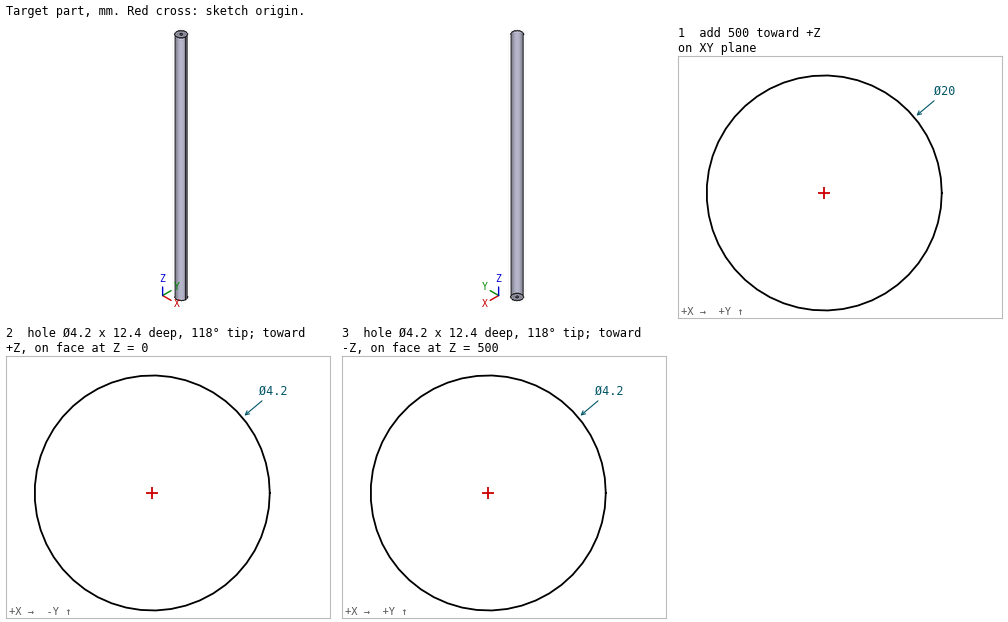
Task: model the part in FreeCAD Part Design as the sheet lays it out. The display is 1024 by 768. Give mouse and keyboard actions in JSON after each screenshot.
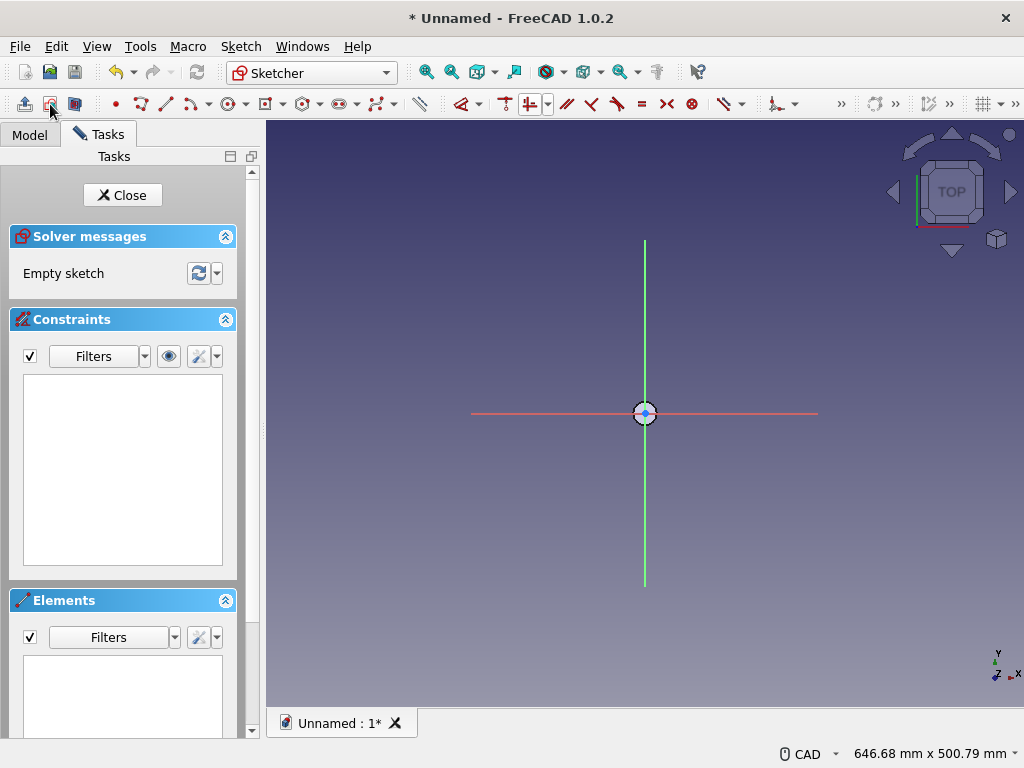
{"action": "scroll", "coordinate": [649, 414], "scroll_direction": "up", "scroll_amount": 15}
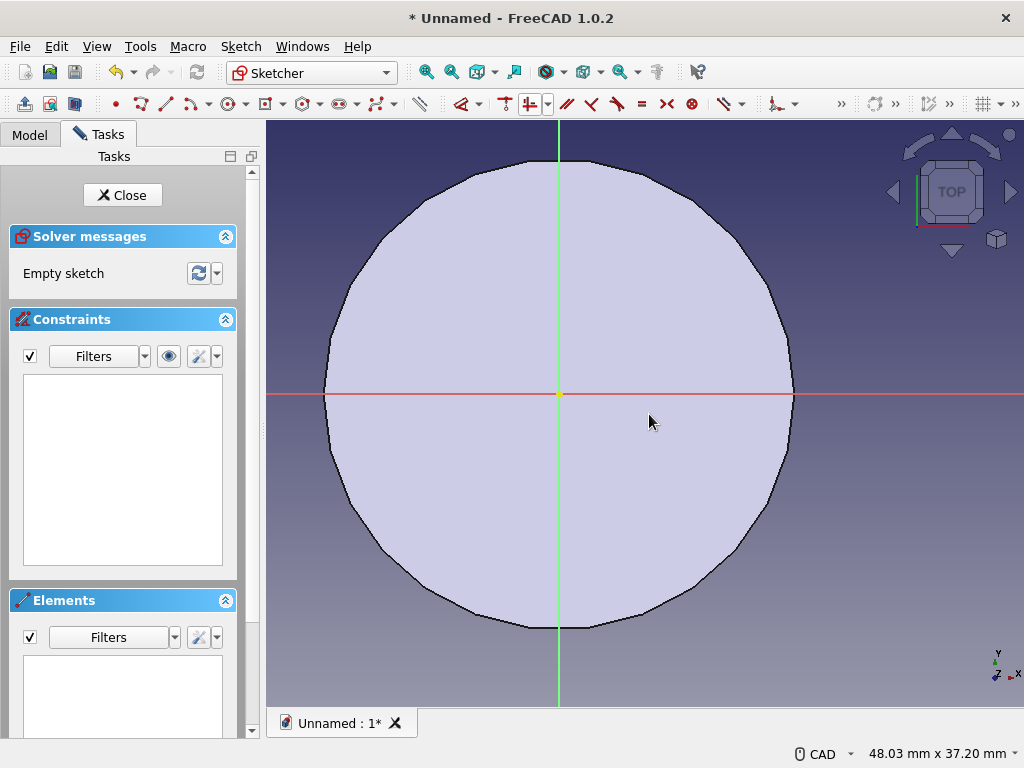
{"action": "scroll", "coordinate": [553, 388], "scroll_direction": "up", "scroll_amount": 7}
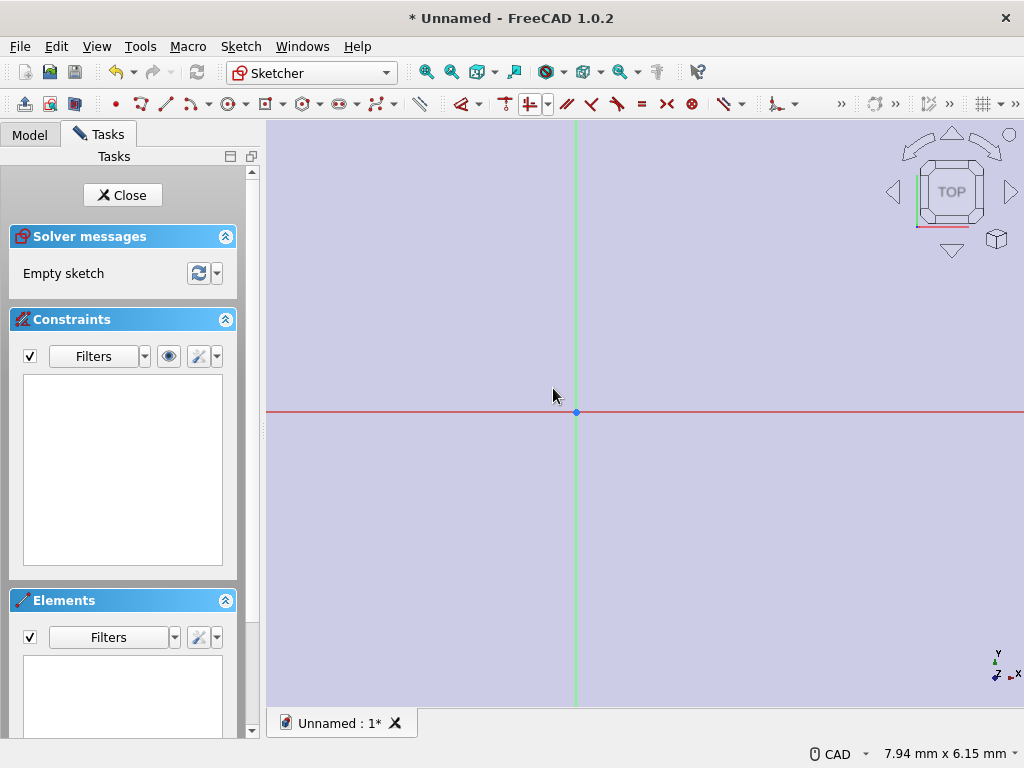
{"action": "key", "text": "g c"}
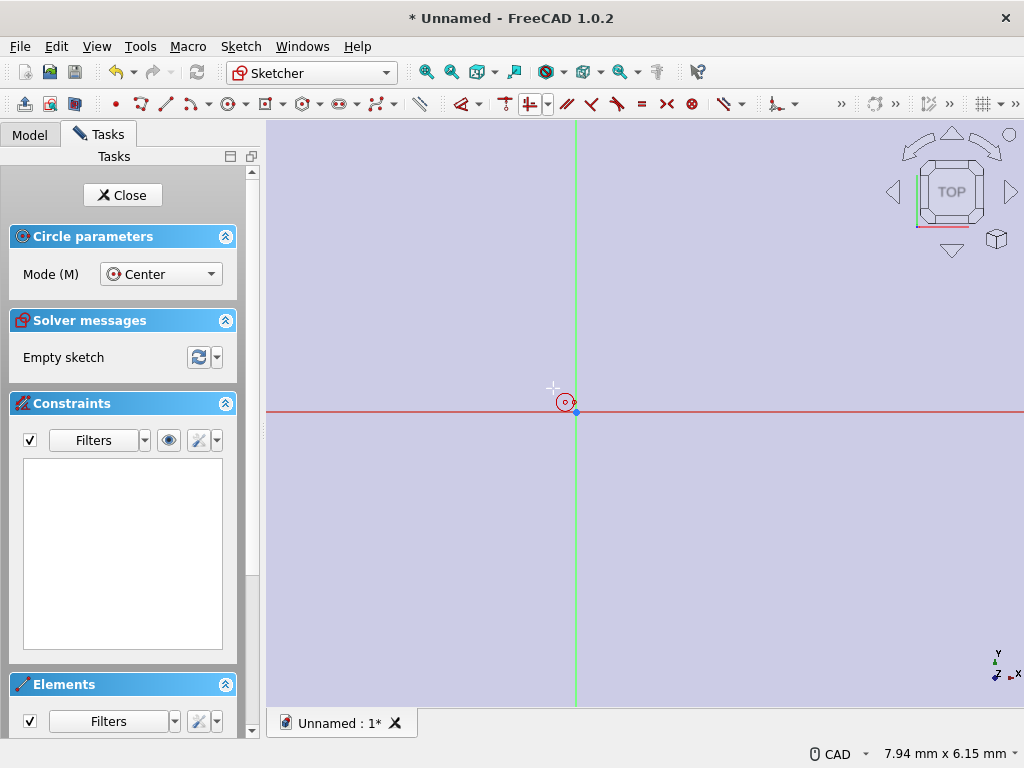
{"action": "left_click", "coordinate": [576, 412]}
{"action": "left_click", "coordinate": [718, 271]}
{"action": "key", "text": "Escape"}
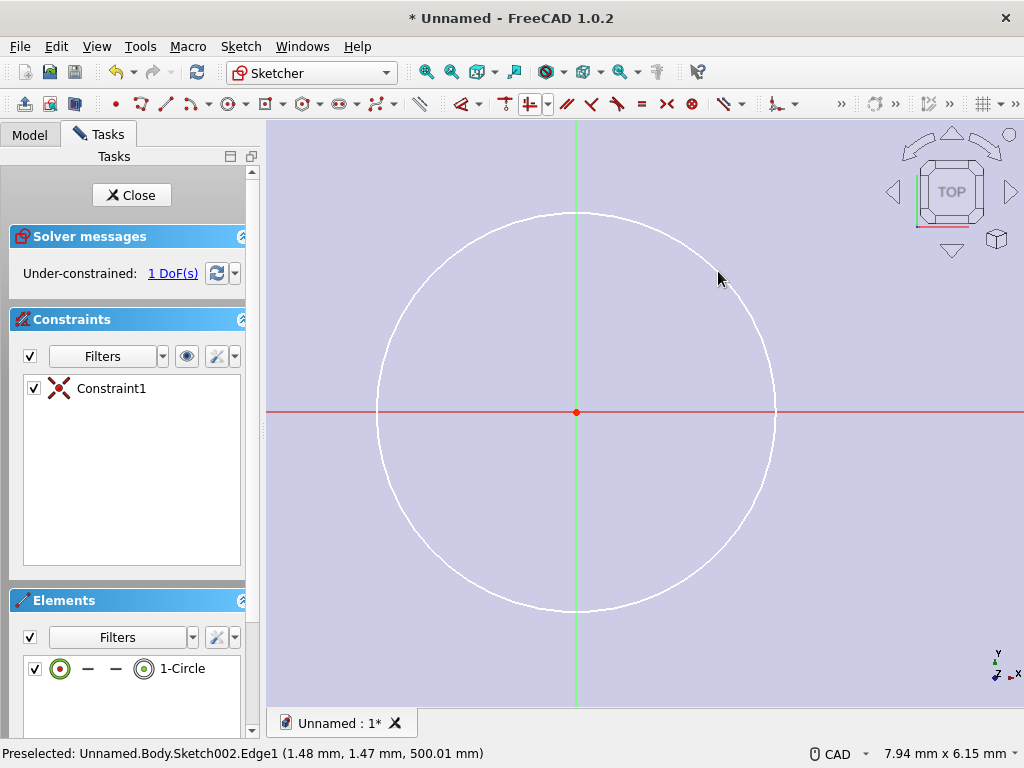
{"action": "left_click", "coordinate": [717, 271]}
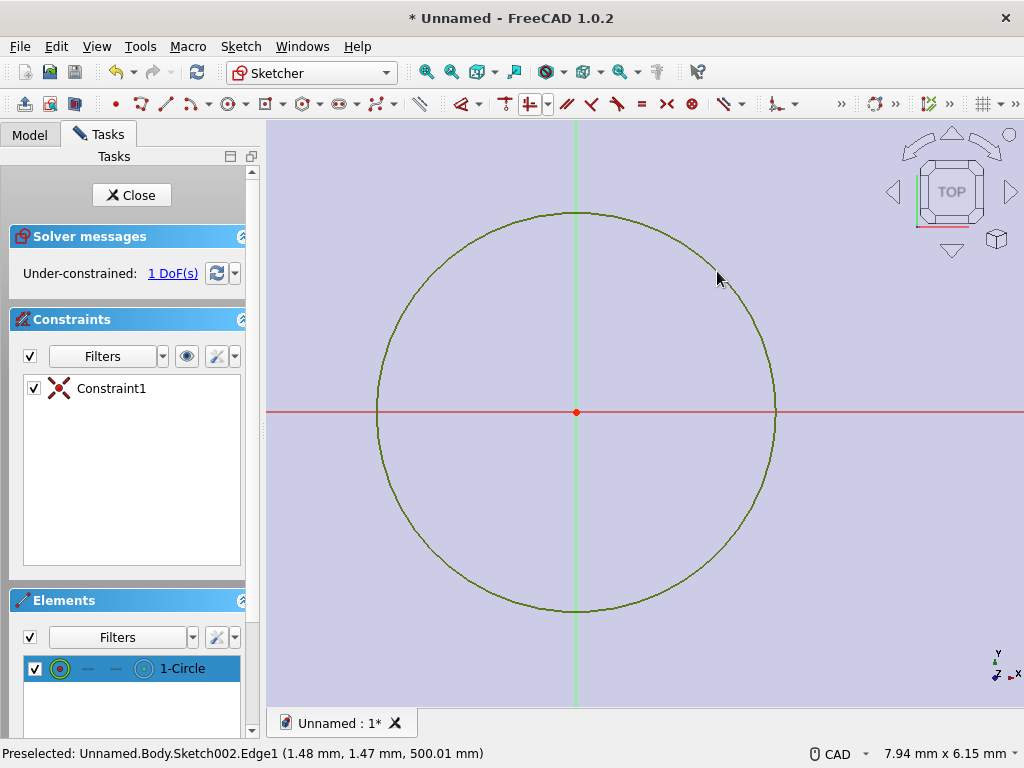
{"action": "left_click", "coordinate": [478, 104]}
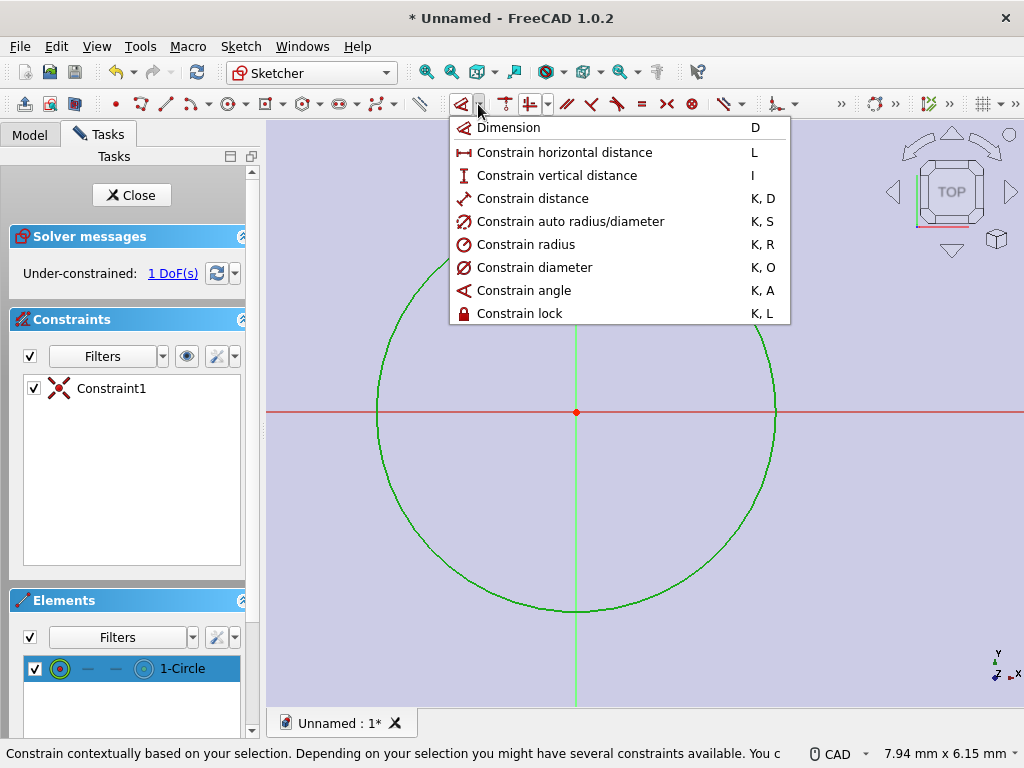
{"action": "left_click", "coordinate": [620, 268]}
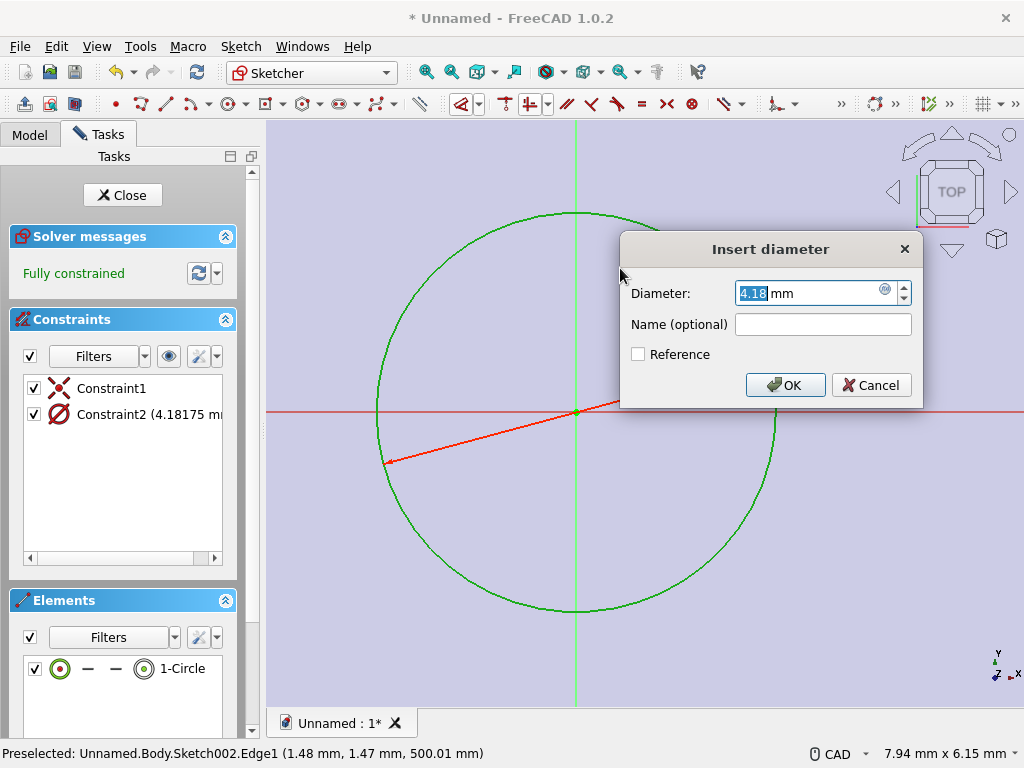
{"action": "type", "text": "4.2"}
{"action": "key", "text": "Return"}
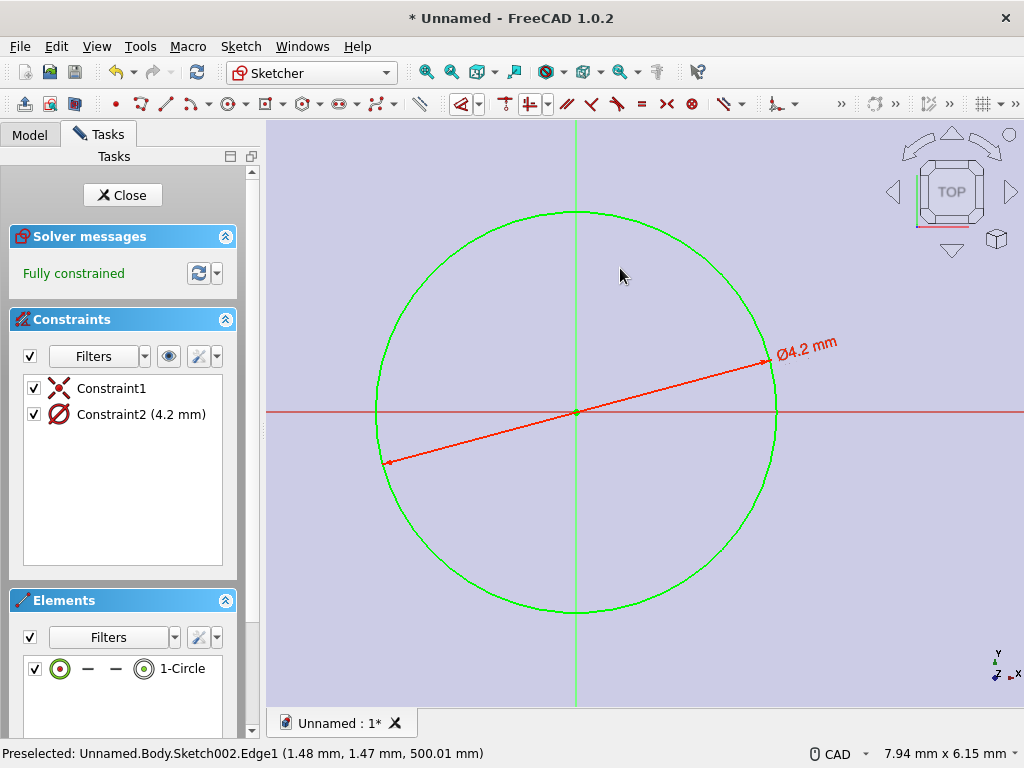
{"action": "left_click", "coordinate": [123, 195]}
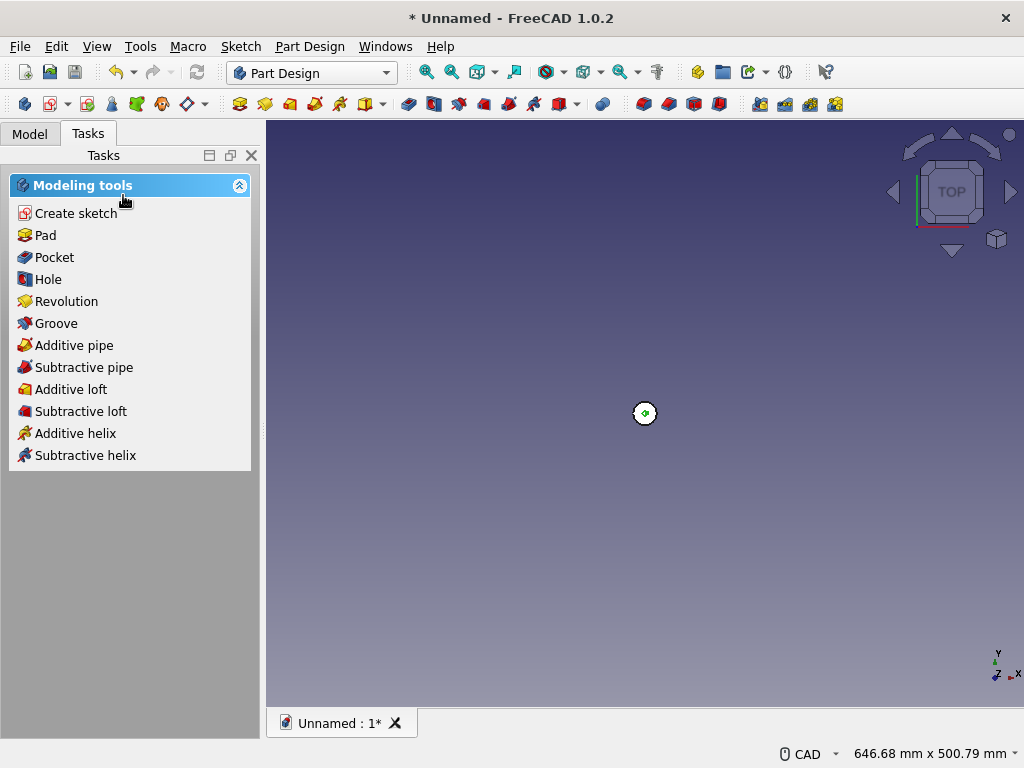
{"action": "left_click", "coordinate": [434, 104]}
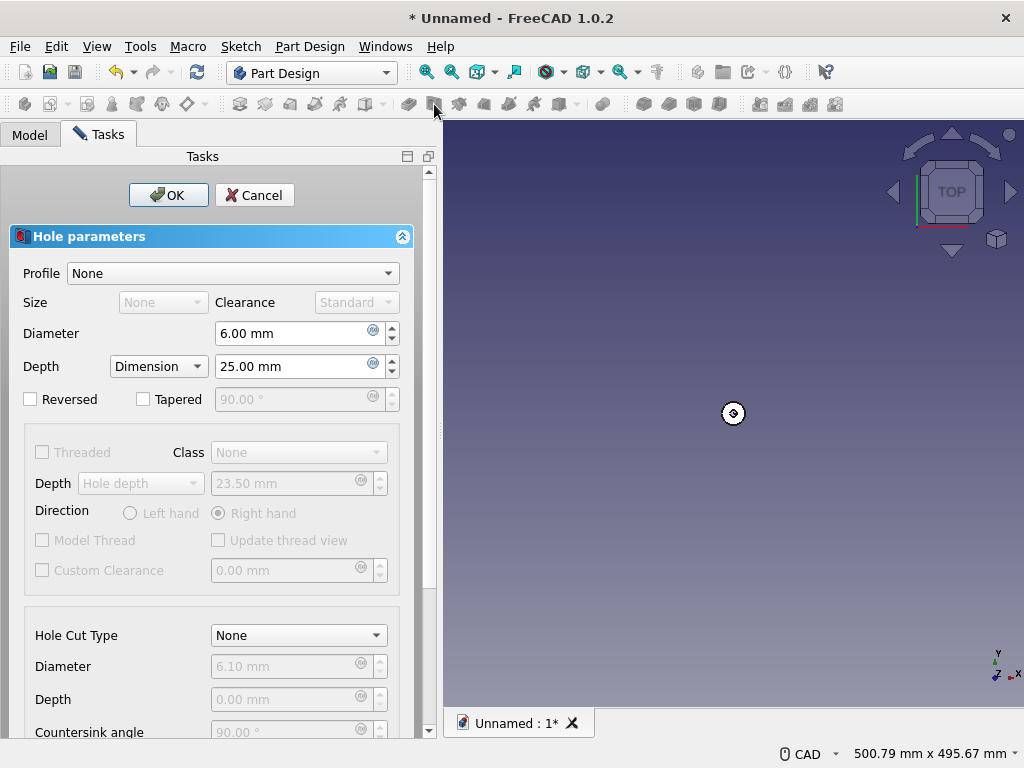
{"action": "triple_click", "coordinate": [300, 334]}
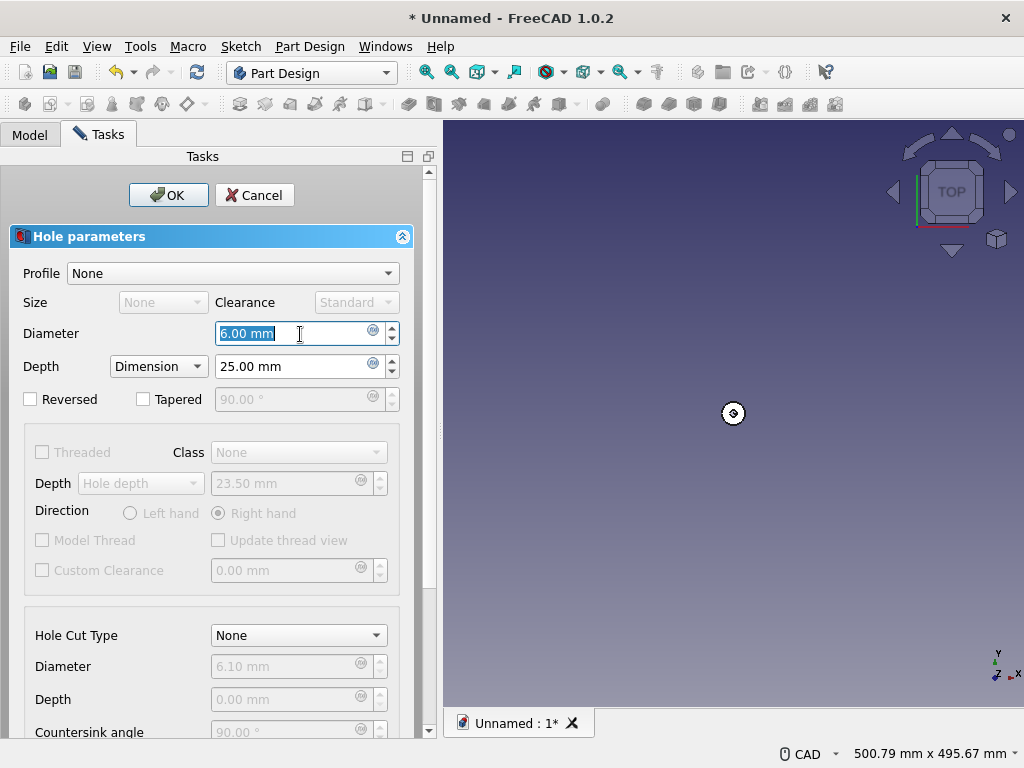
{"action": "type", "text": "4.2"}
{"action": "key", "text": "Tab"}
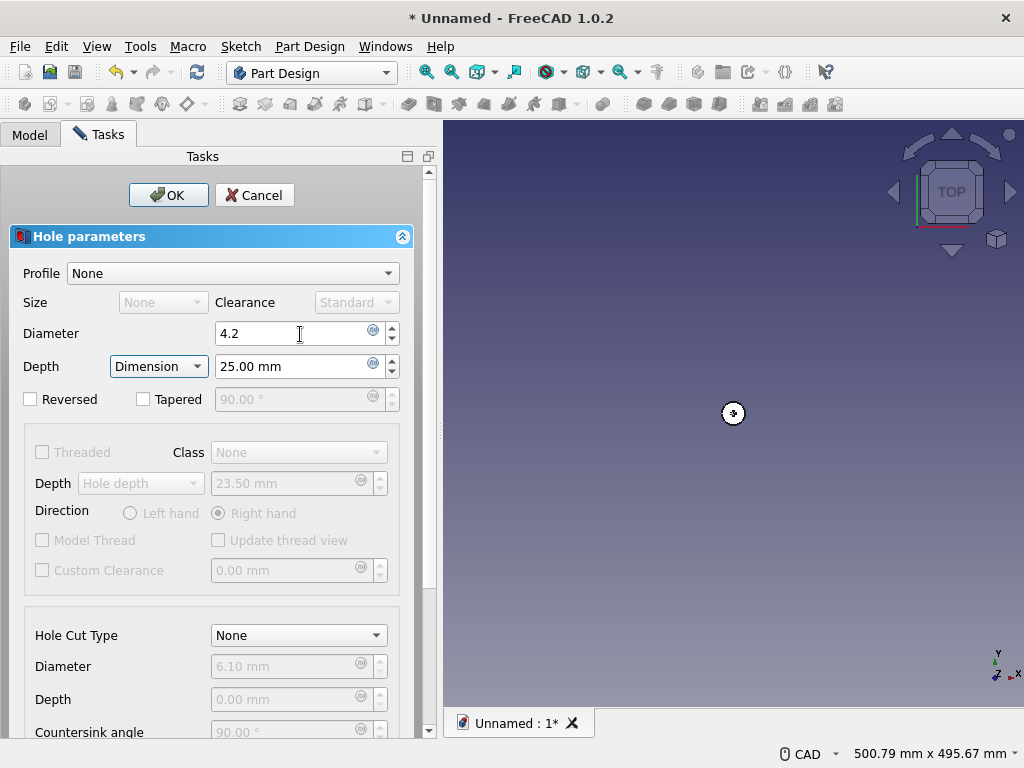
{"action": "triple_click", "coordinate": [300, 366]}